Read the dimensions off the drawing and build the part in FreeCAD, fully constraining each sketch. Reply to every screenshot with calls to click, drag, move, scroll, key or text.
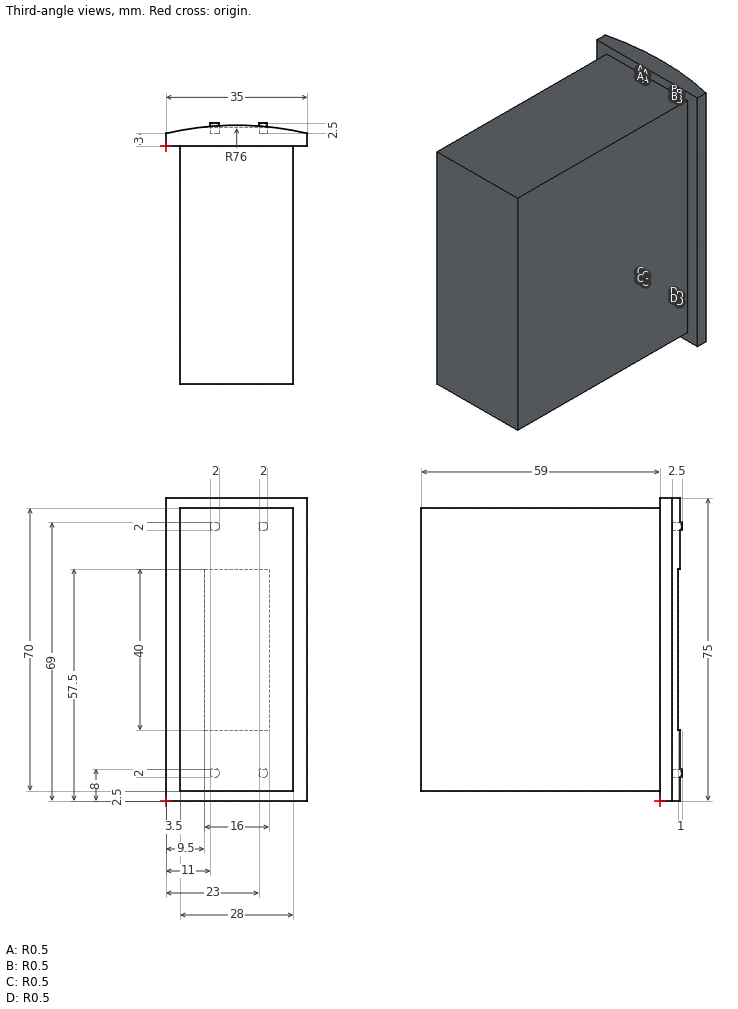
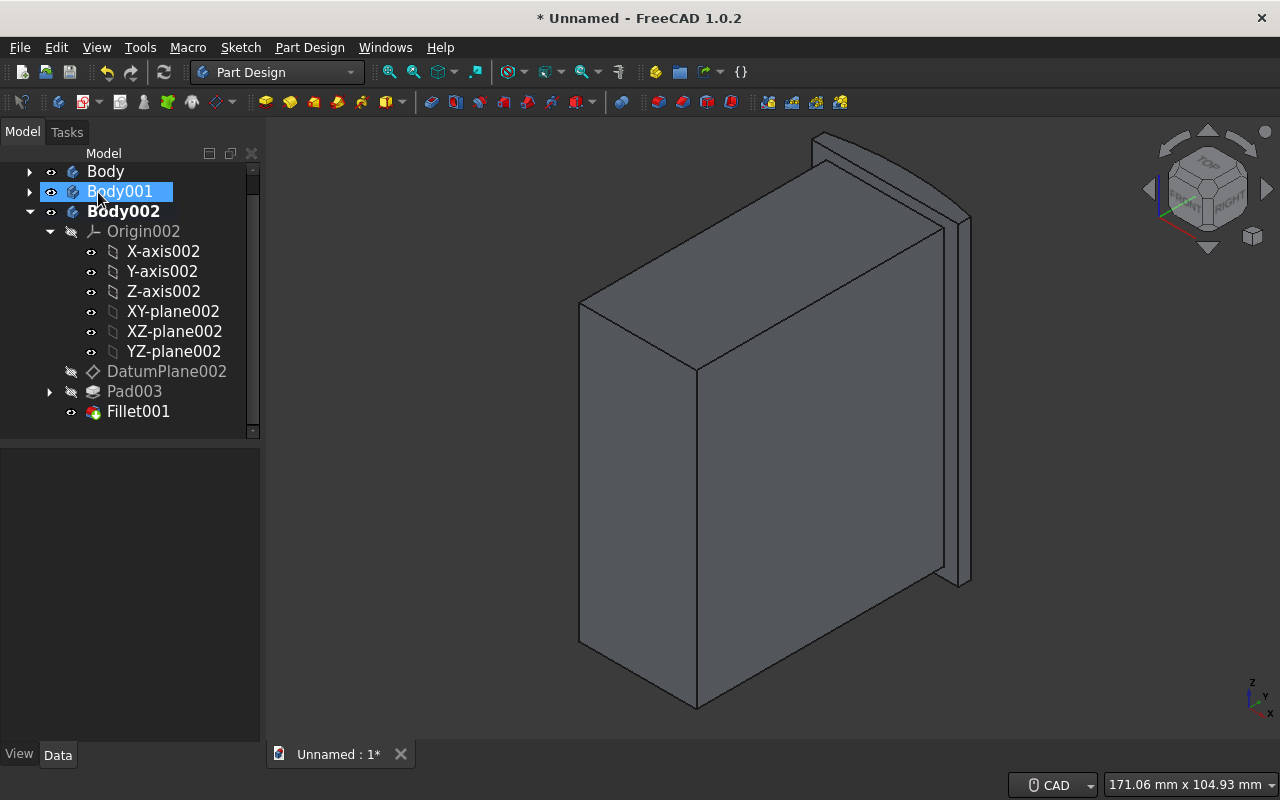
click(60, 102)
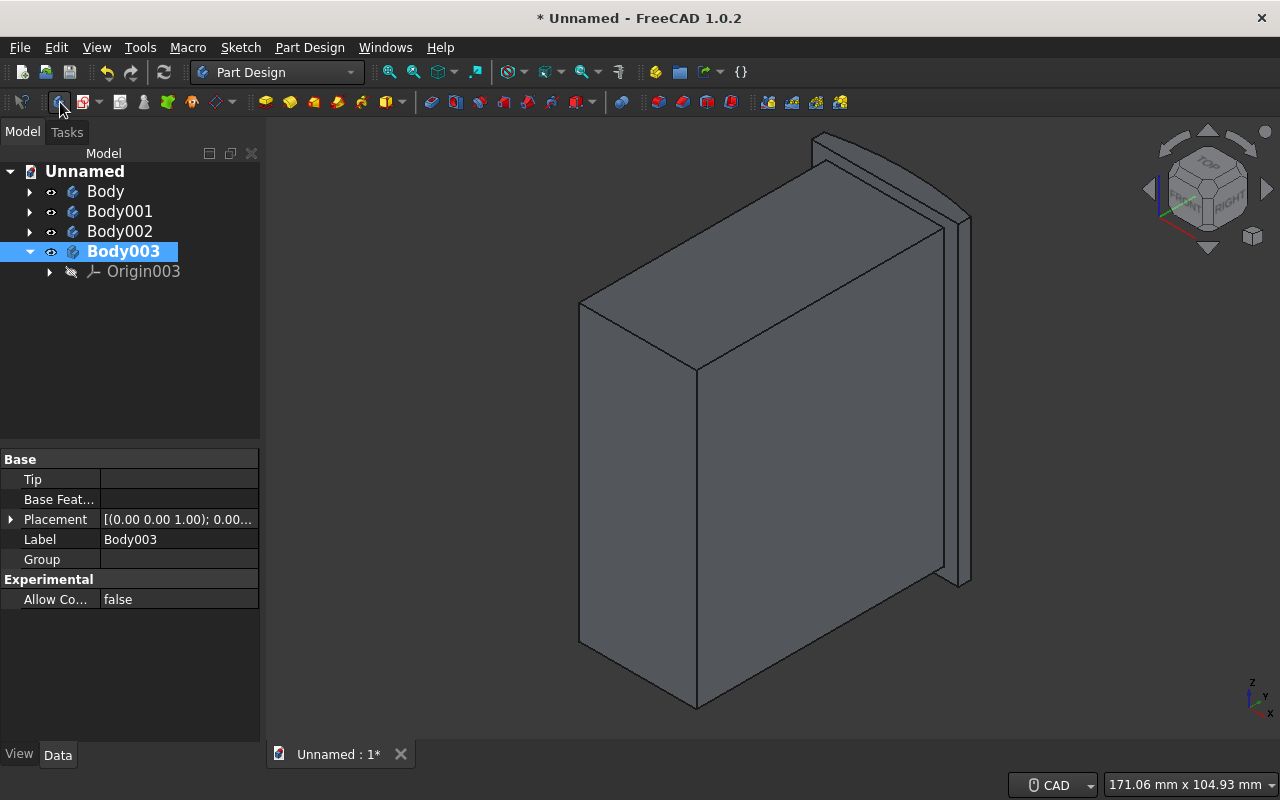
click(50, 272)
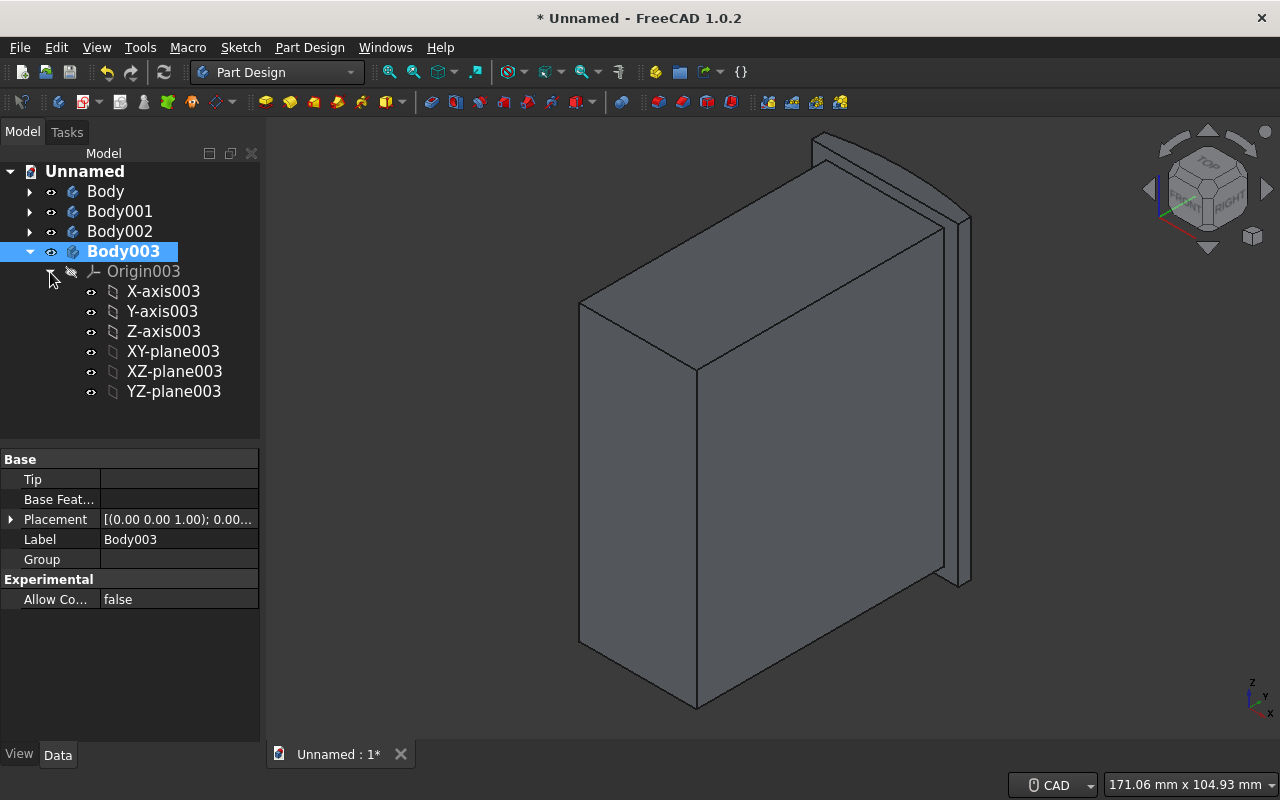
click(136, 372)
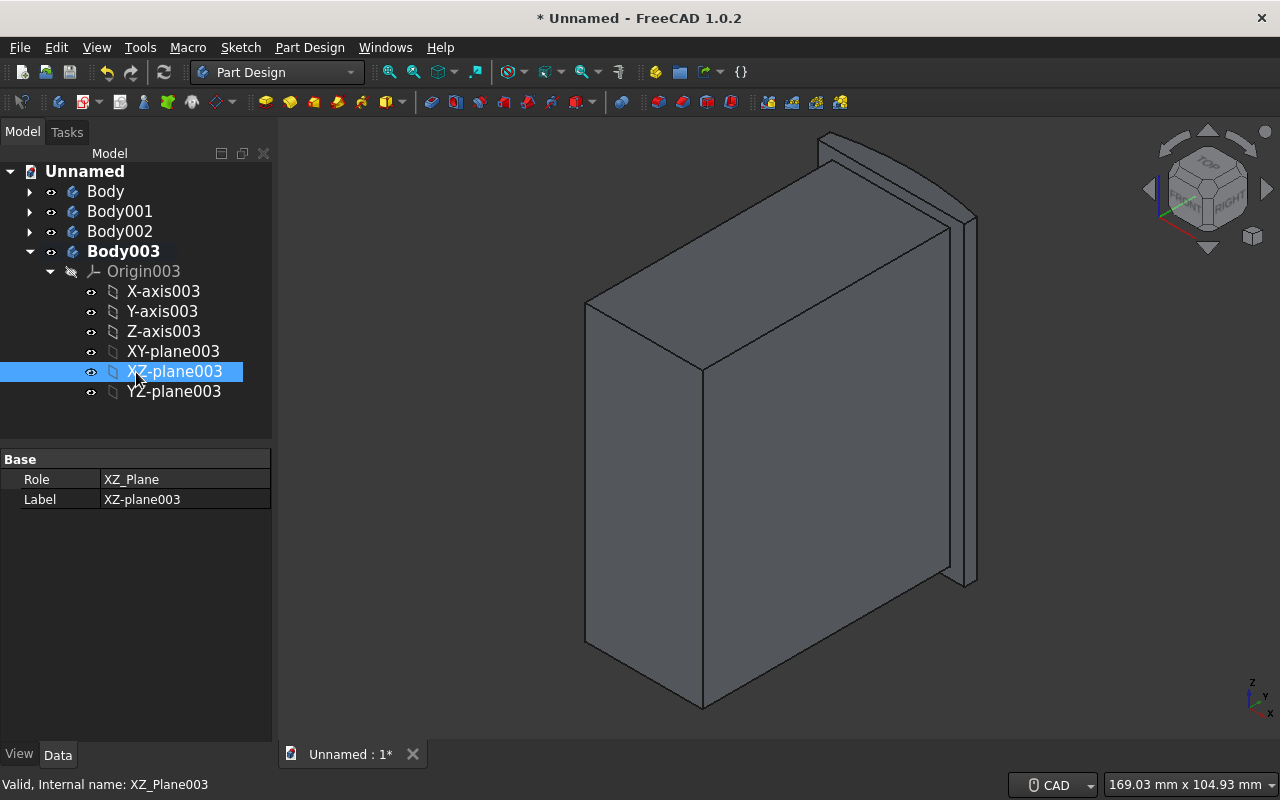
click(216, 102)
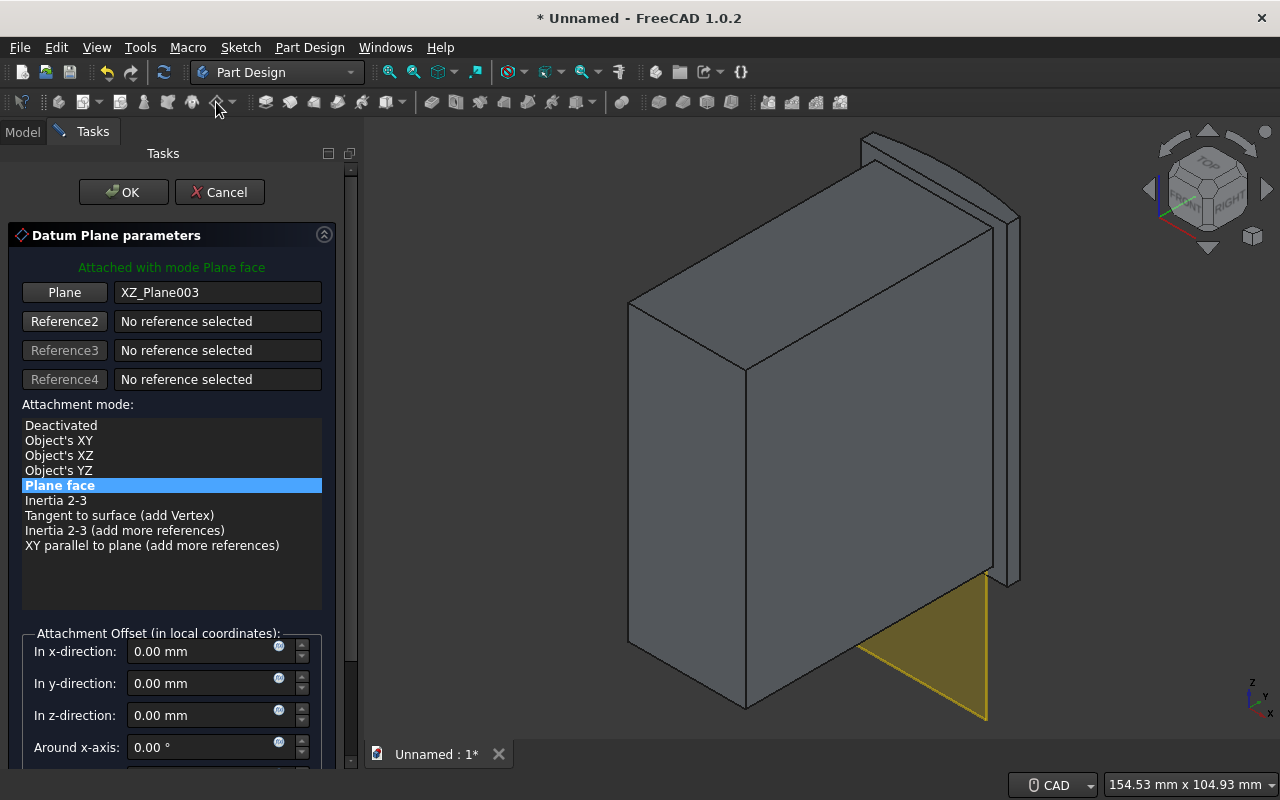
triple_click(210, 715)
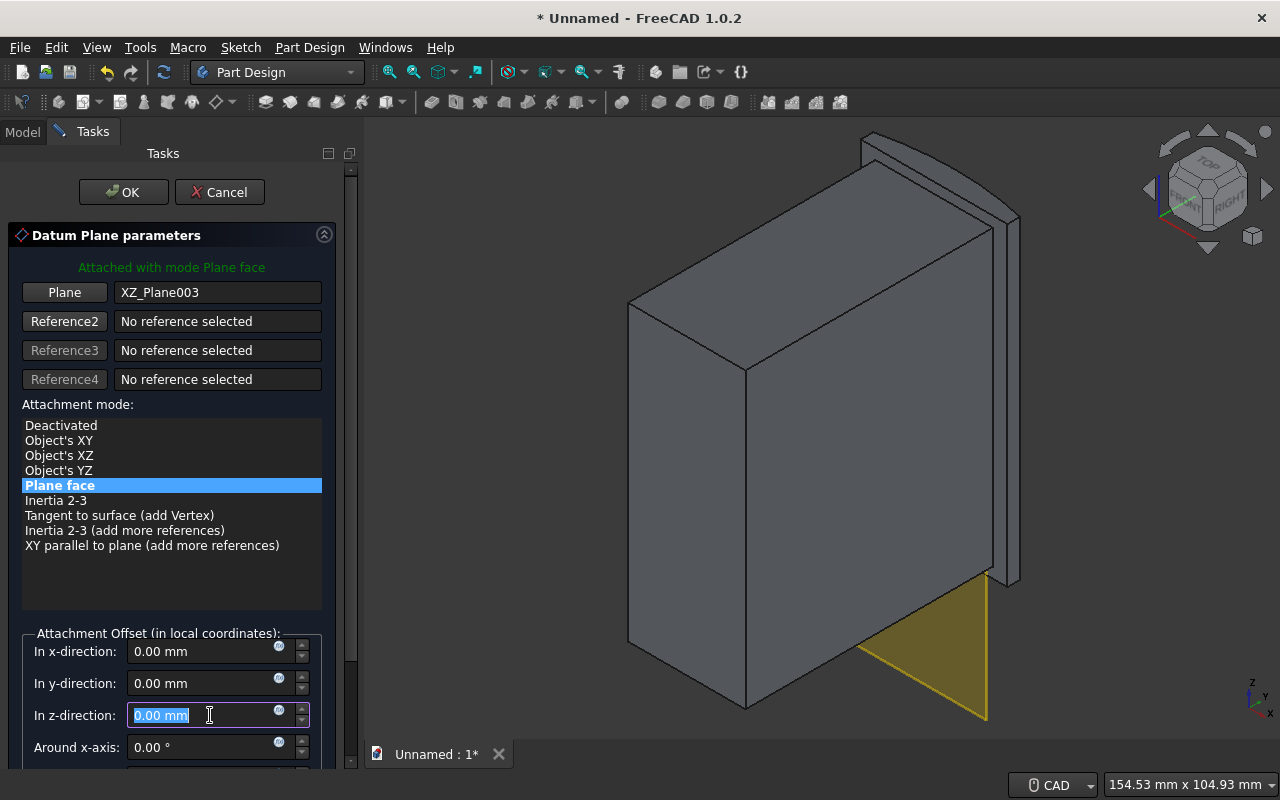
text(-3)
key(Tab)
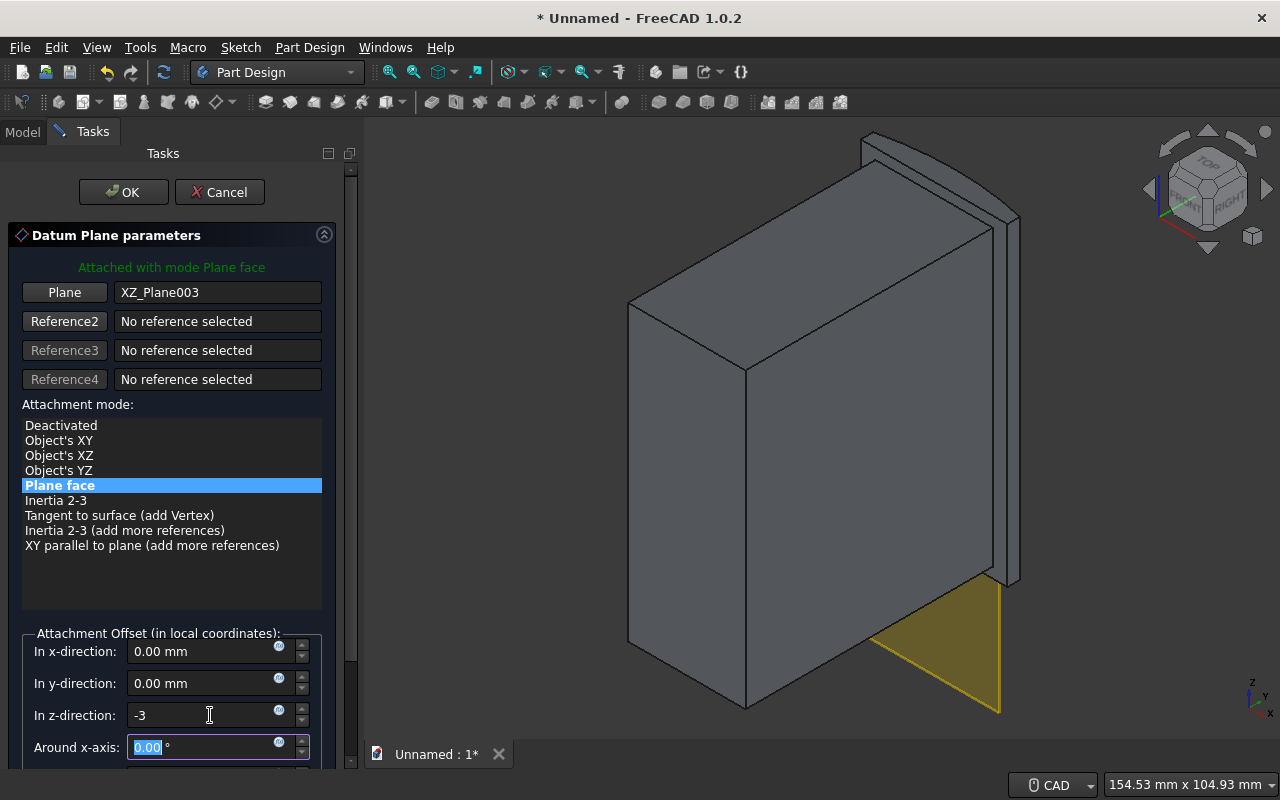
click(124, 192)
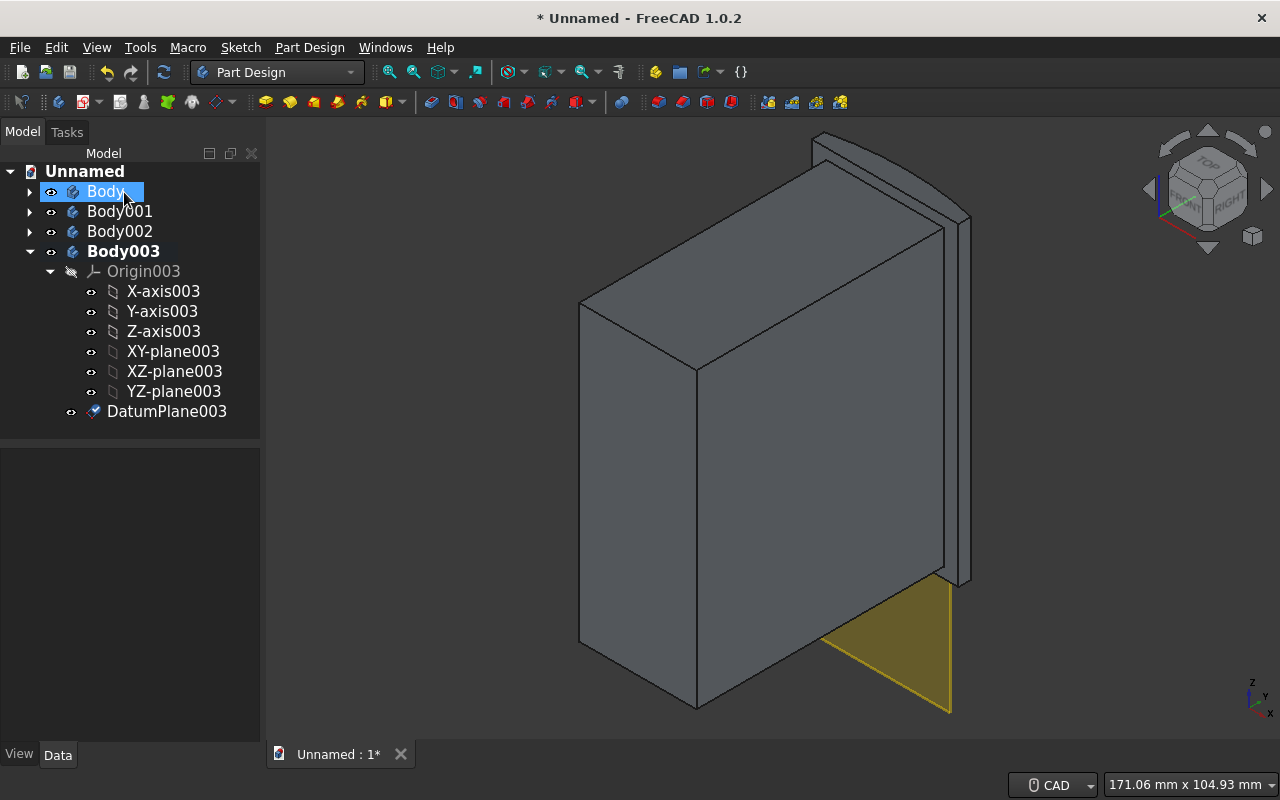
click(116, 412)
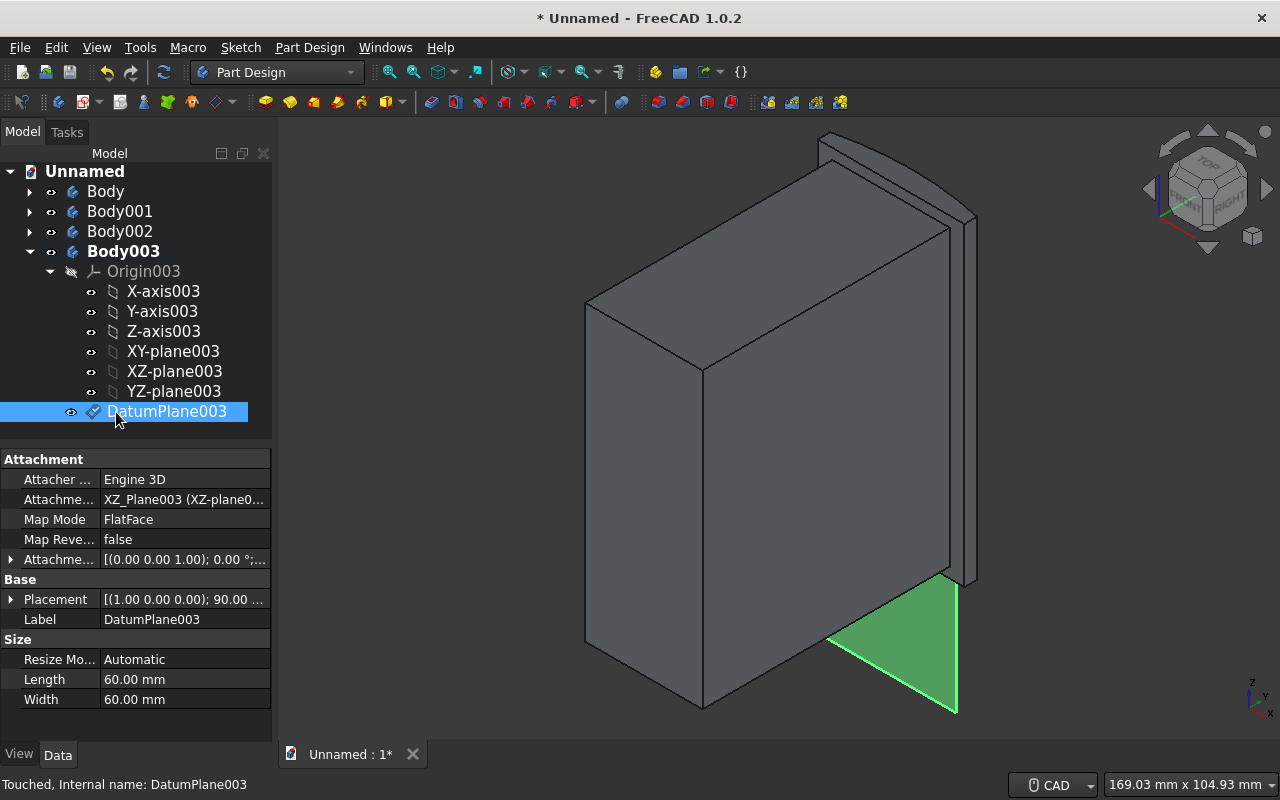
click(84, 102)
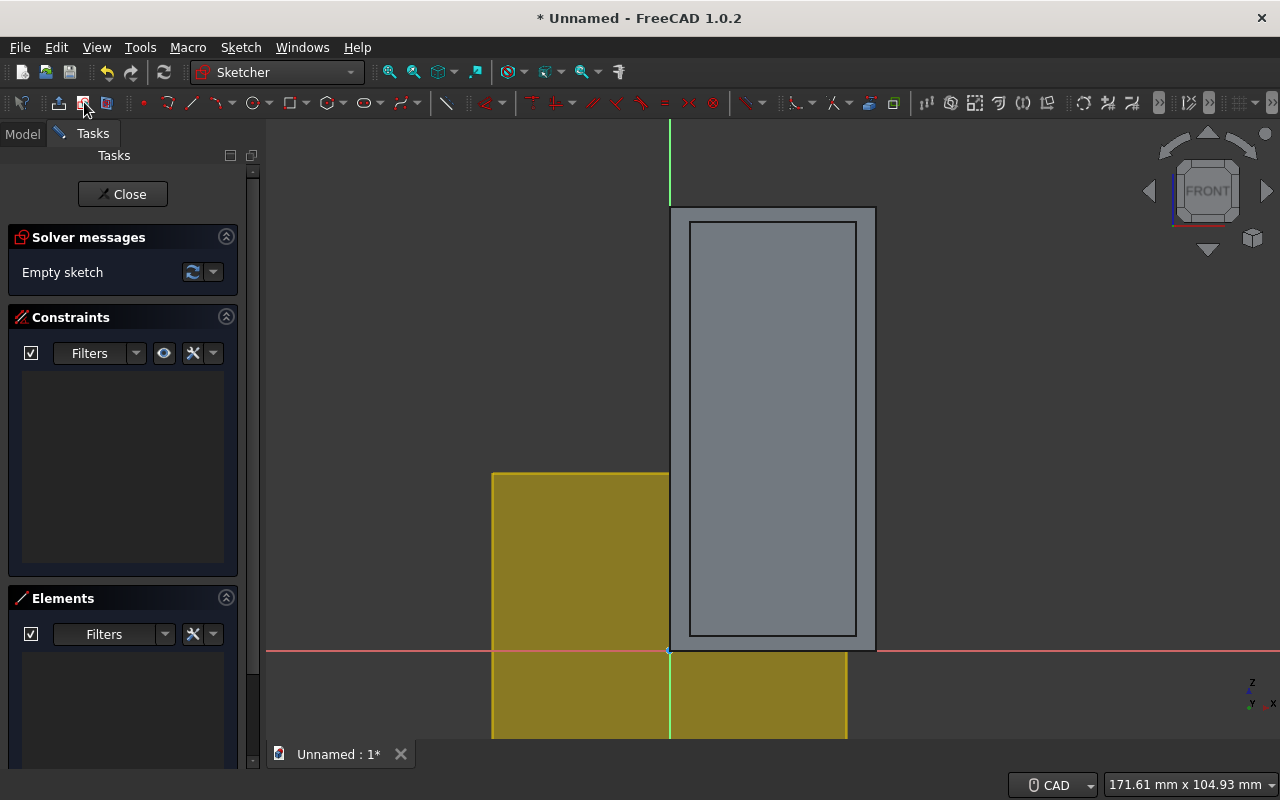
scroll(742, 619, up, 15)